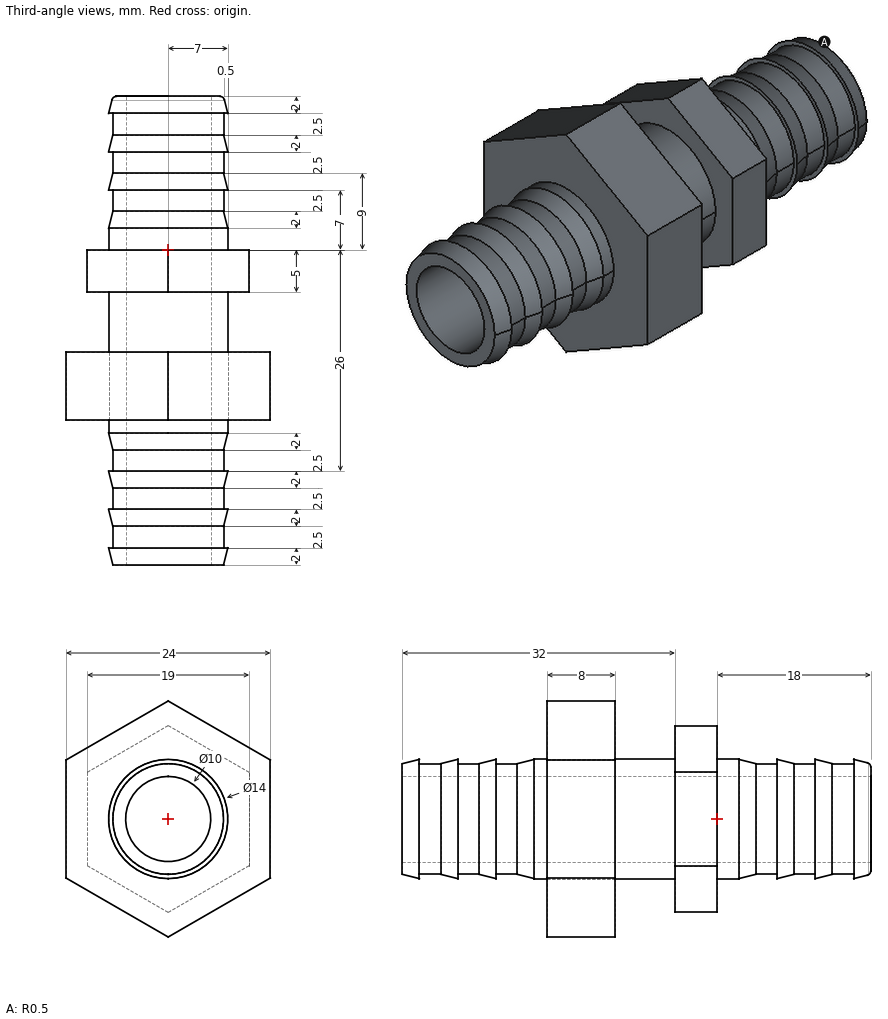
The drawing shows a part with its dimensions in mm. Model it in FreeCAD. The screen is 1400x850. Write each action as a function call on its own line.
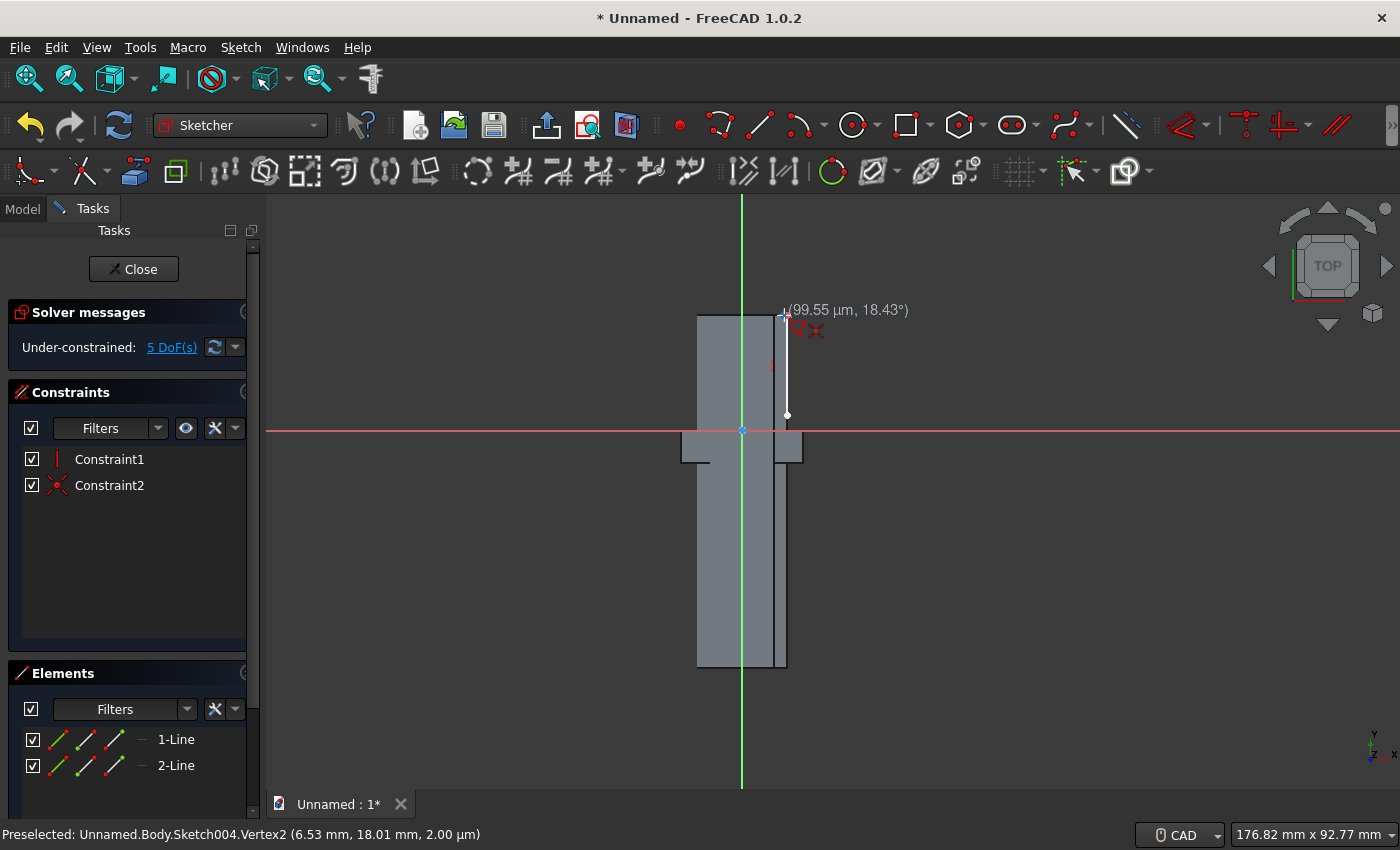
scroll(787, 328, up, 2)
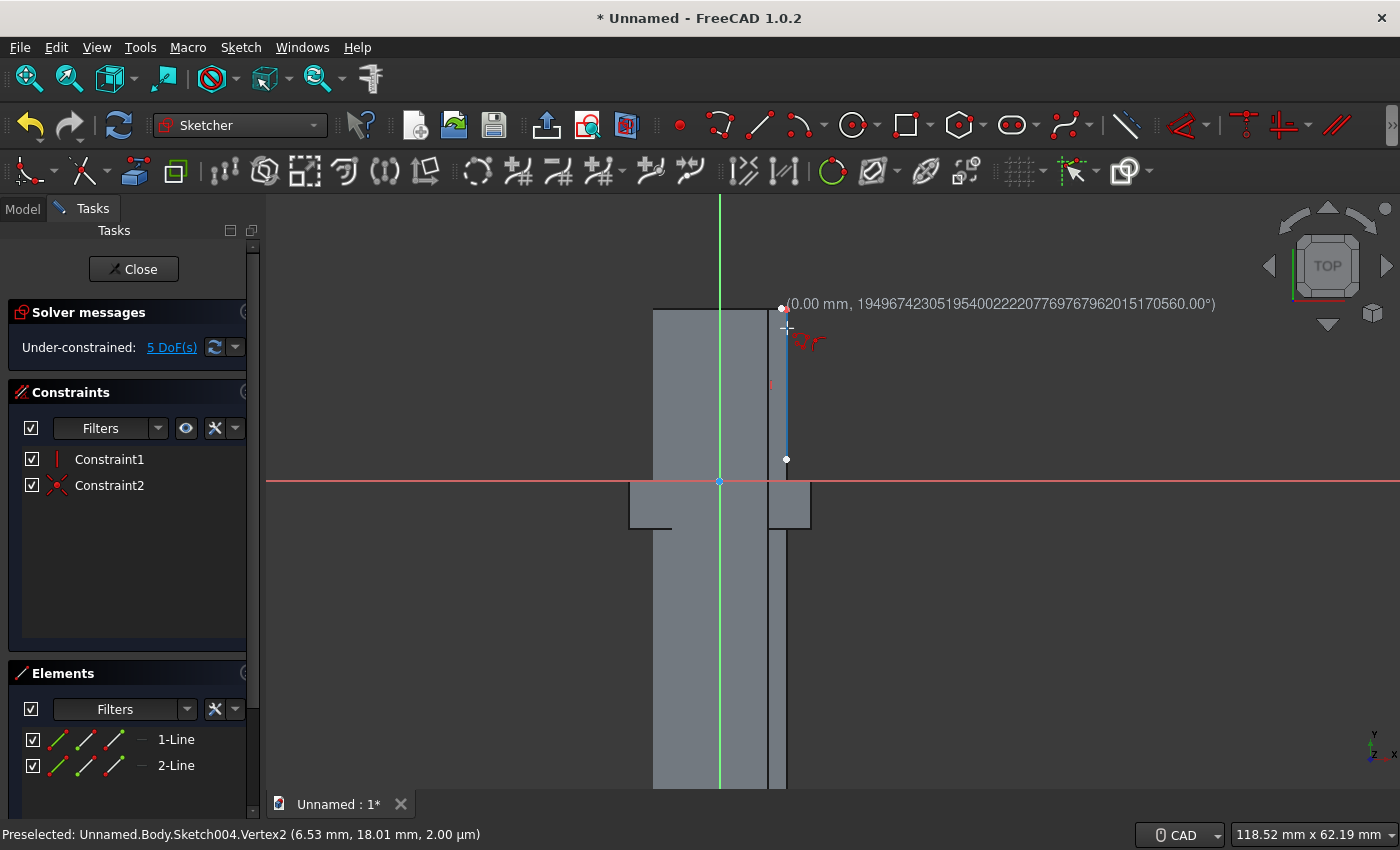
click(787, 328)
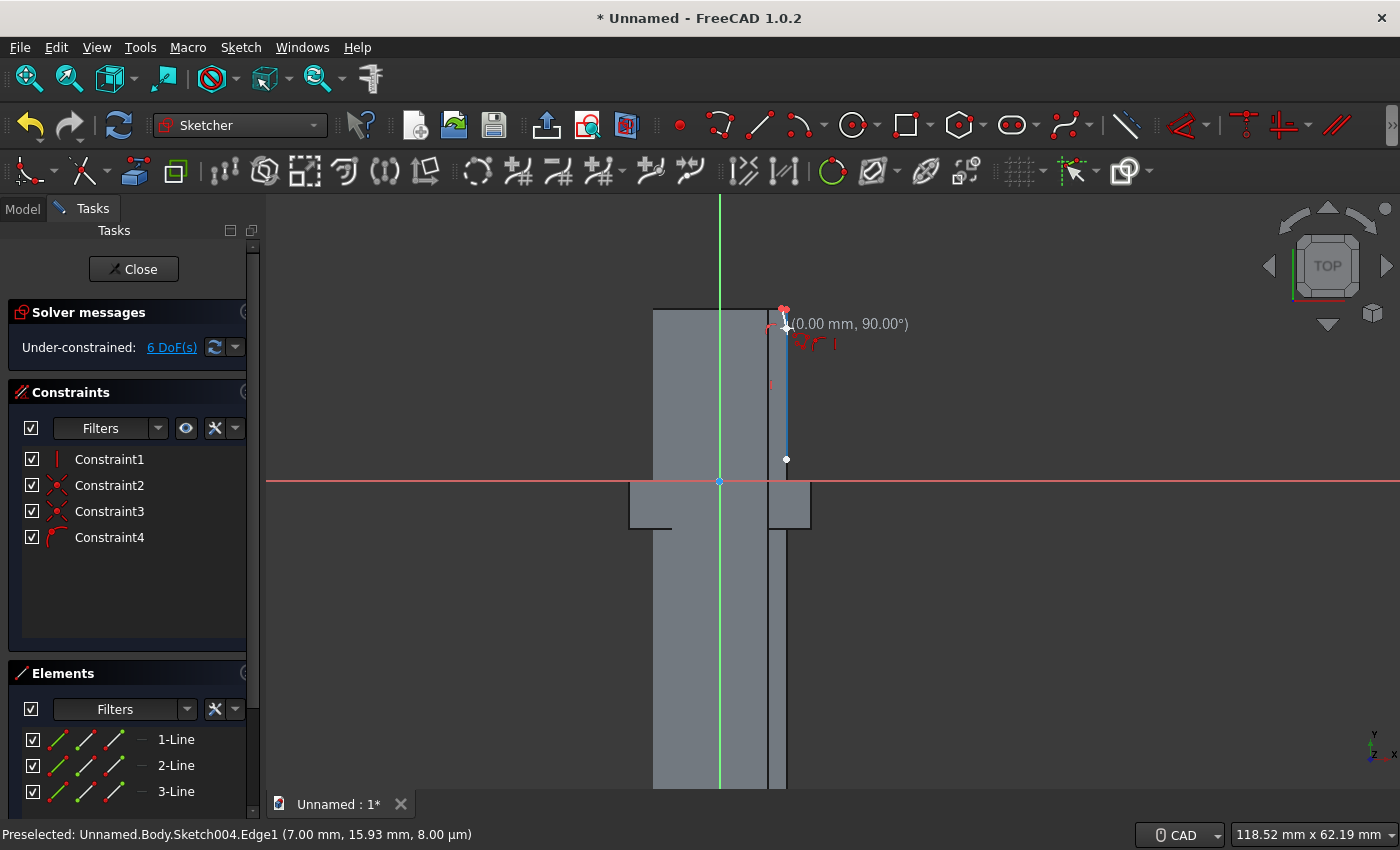
scroll(782, 328, up, 7)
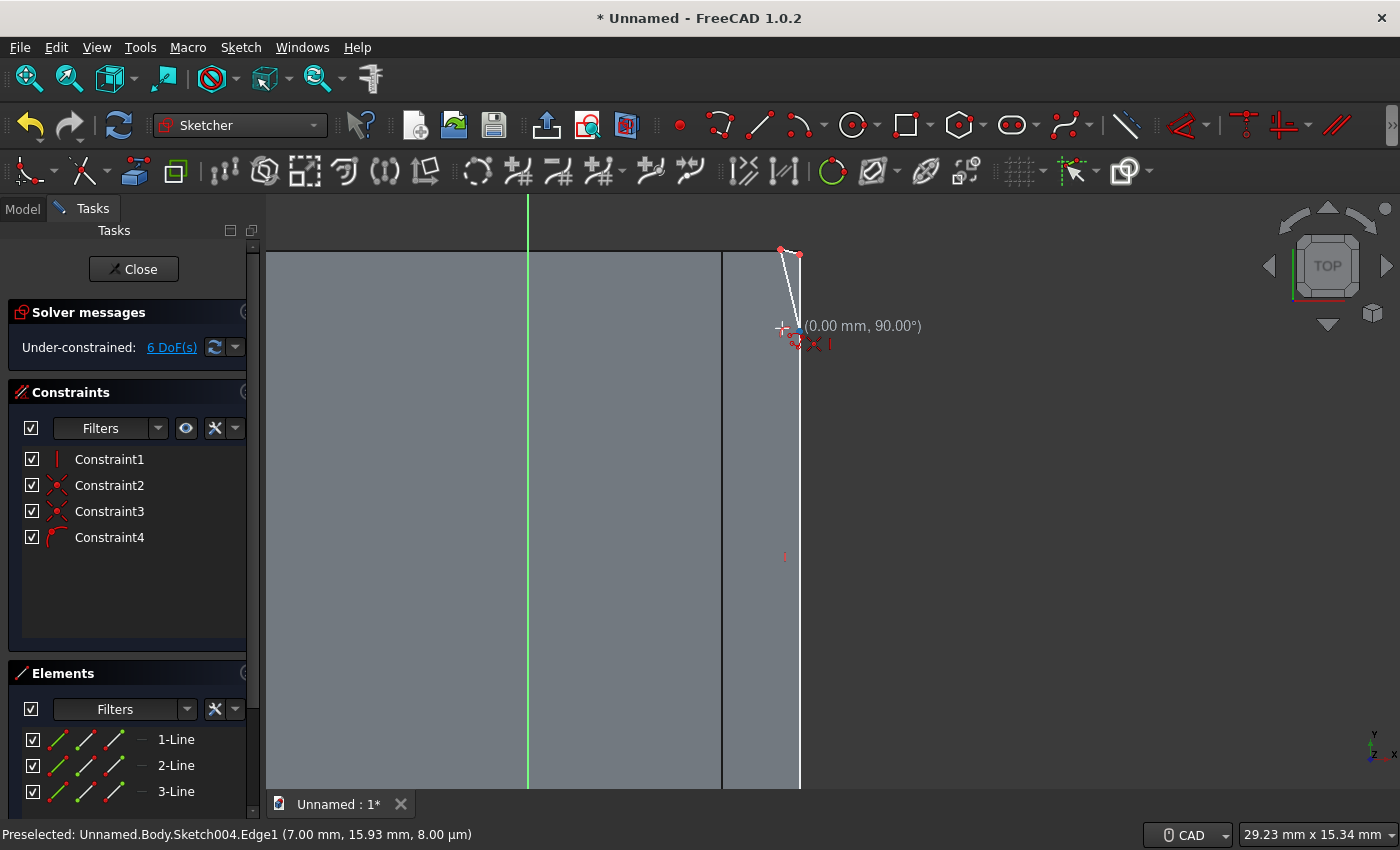
click(780, 327)
click(780, 426)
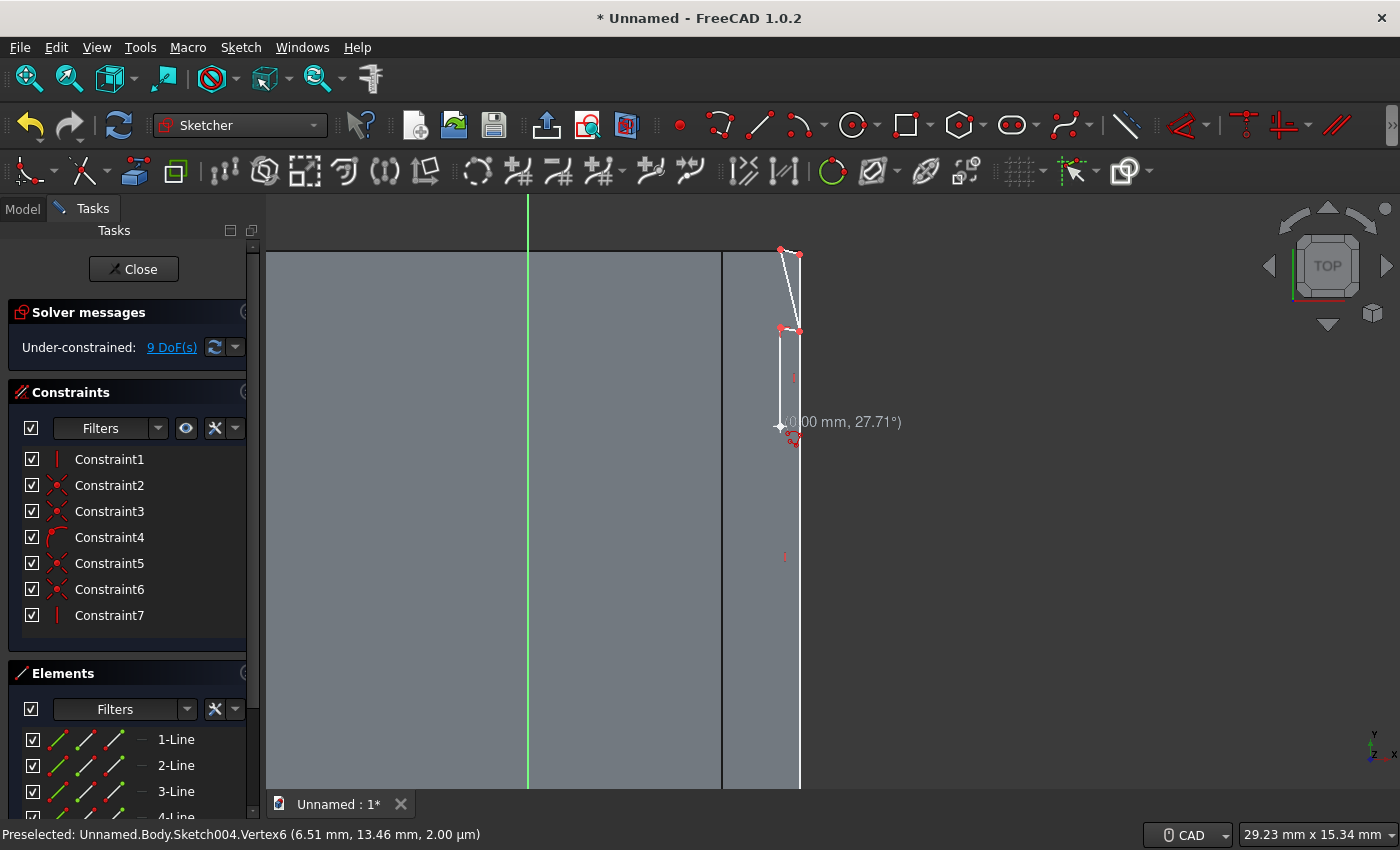
scroll(784, 328, down, 9)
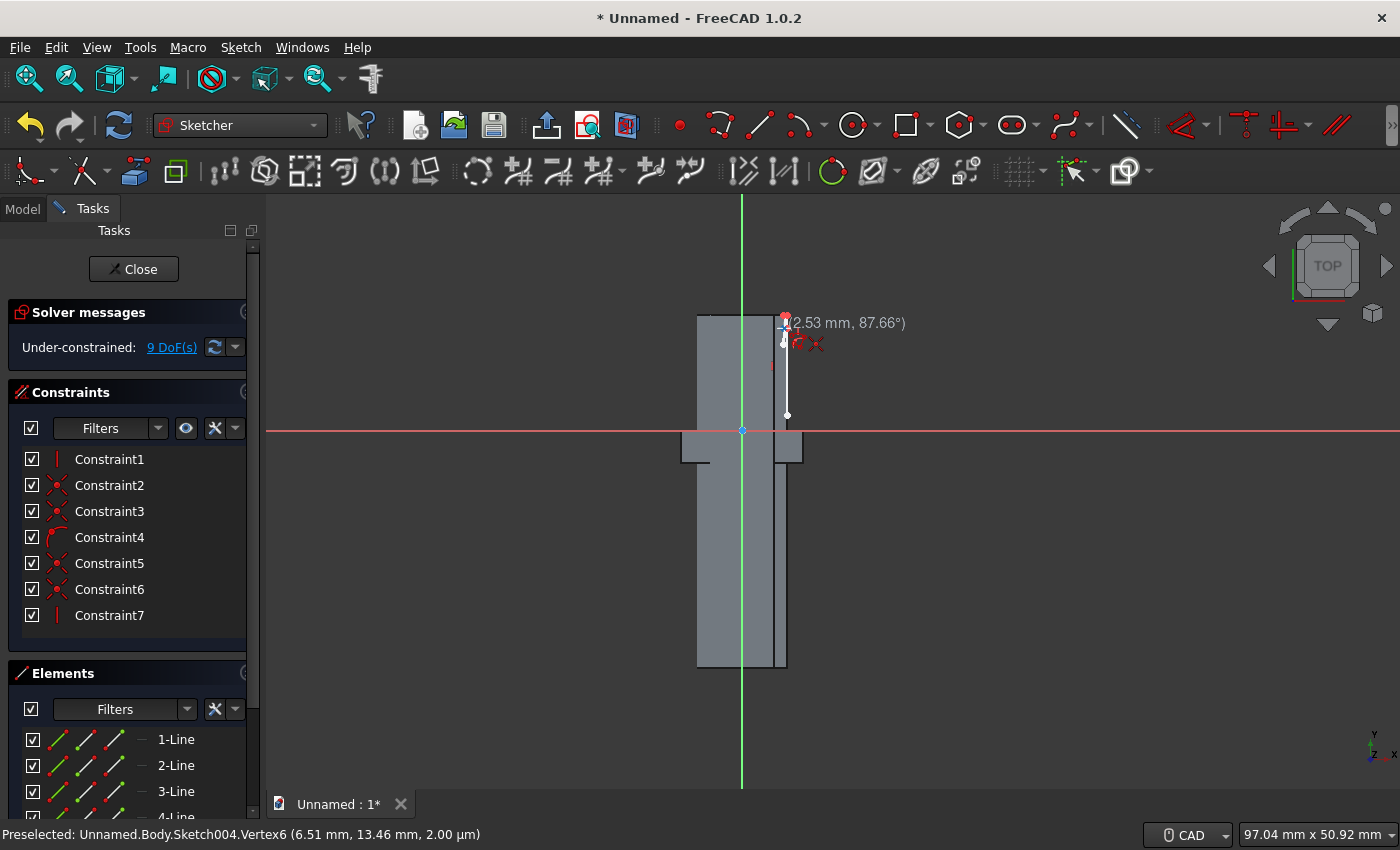
scroll(787, 357, up, 4)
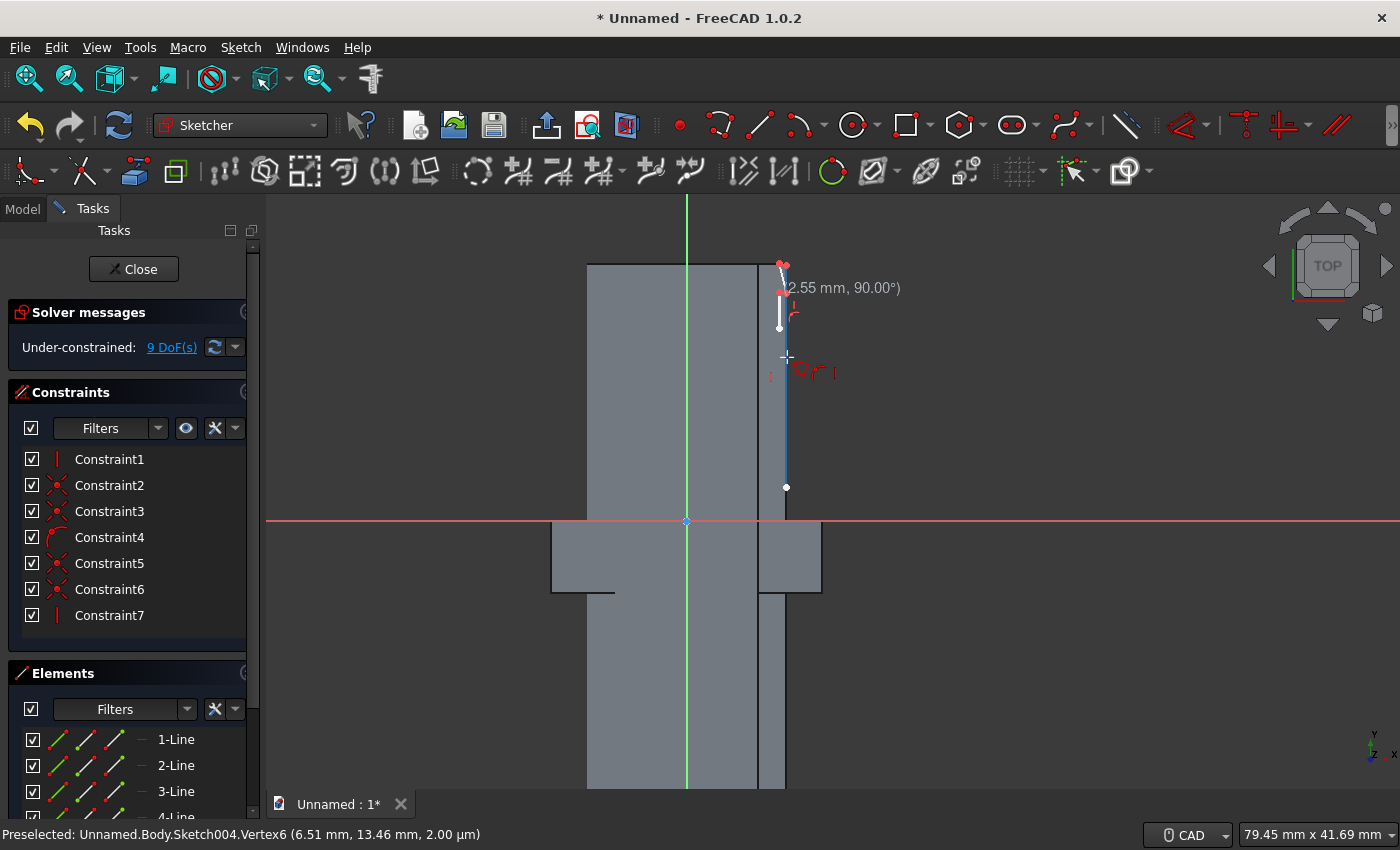
click(786, 357)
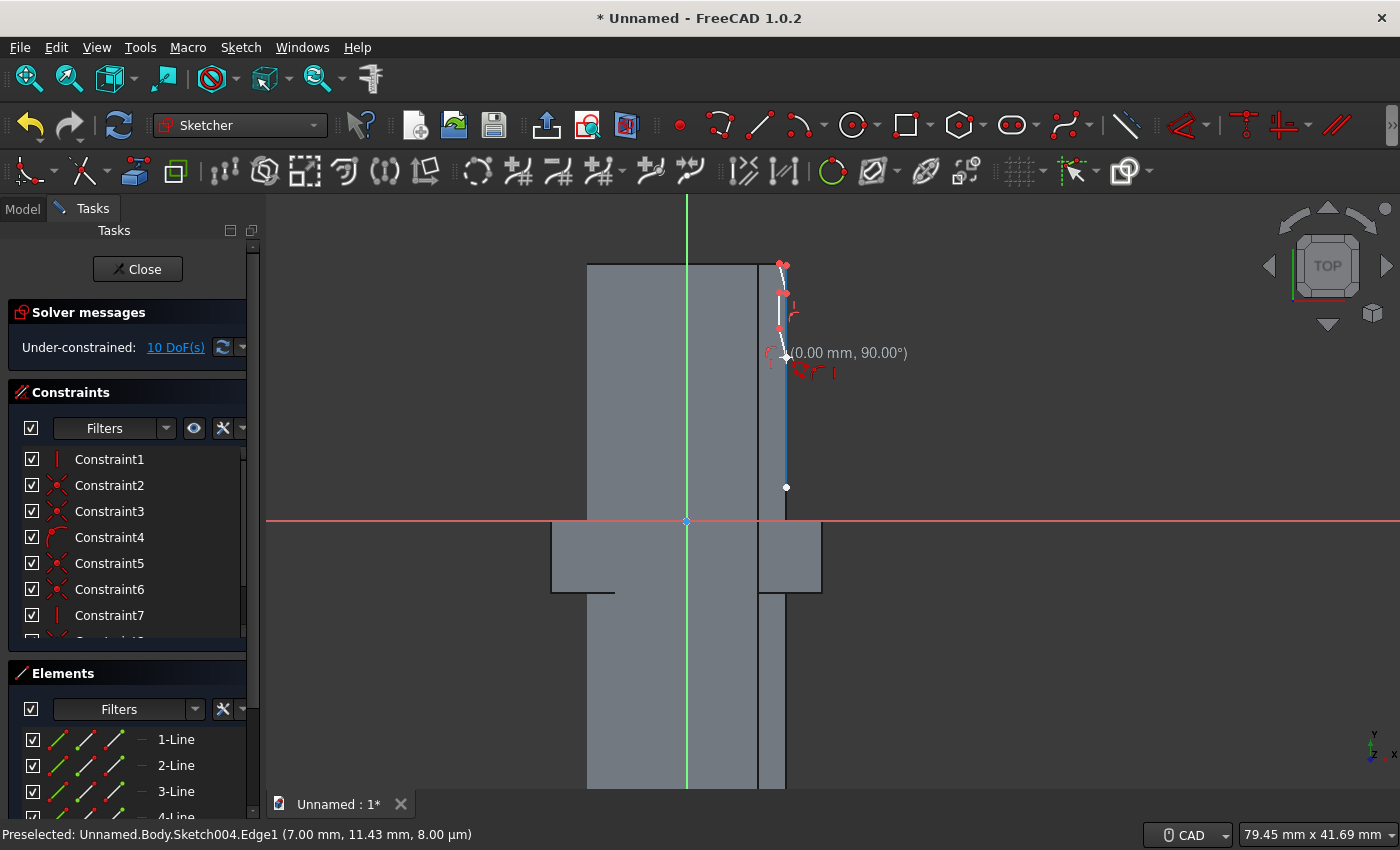
scroll(779, 357, up, 5)